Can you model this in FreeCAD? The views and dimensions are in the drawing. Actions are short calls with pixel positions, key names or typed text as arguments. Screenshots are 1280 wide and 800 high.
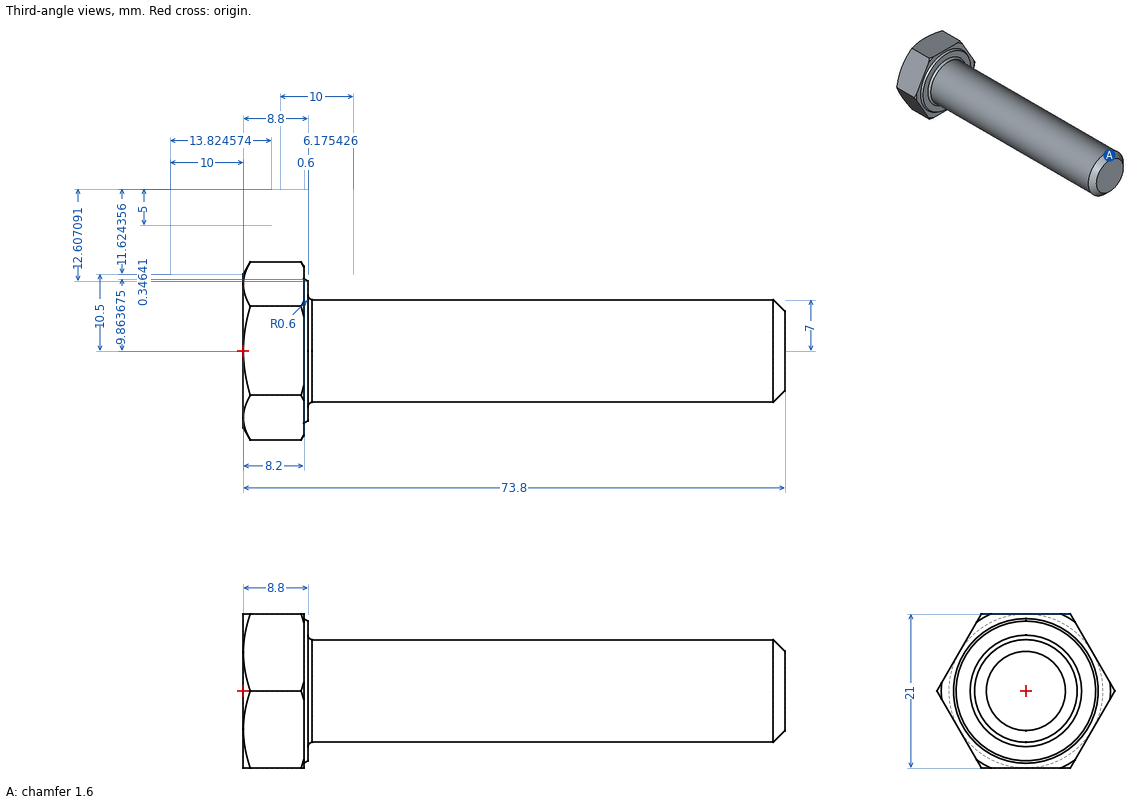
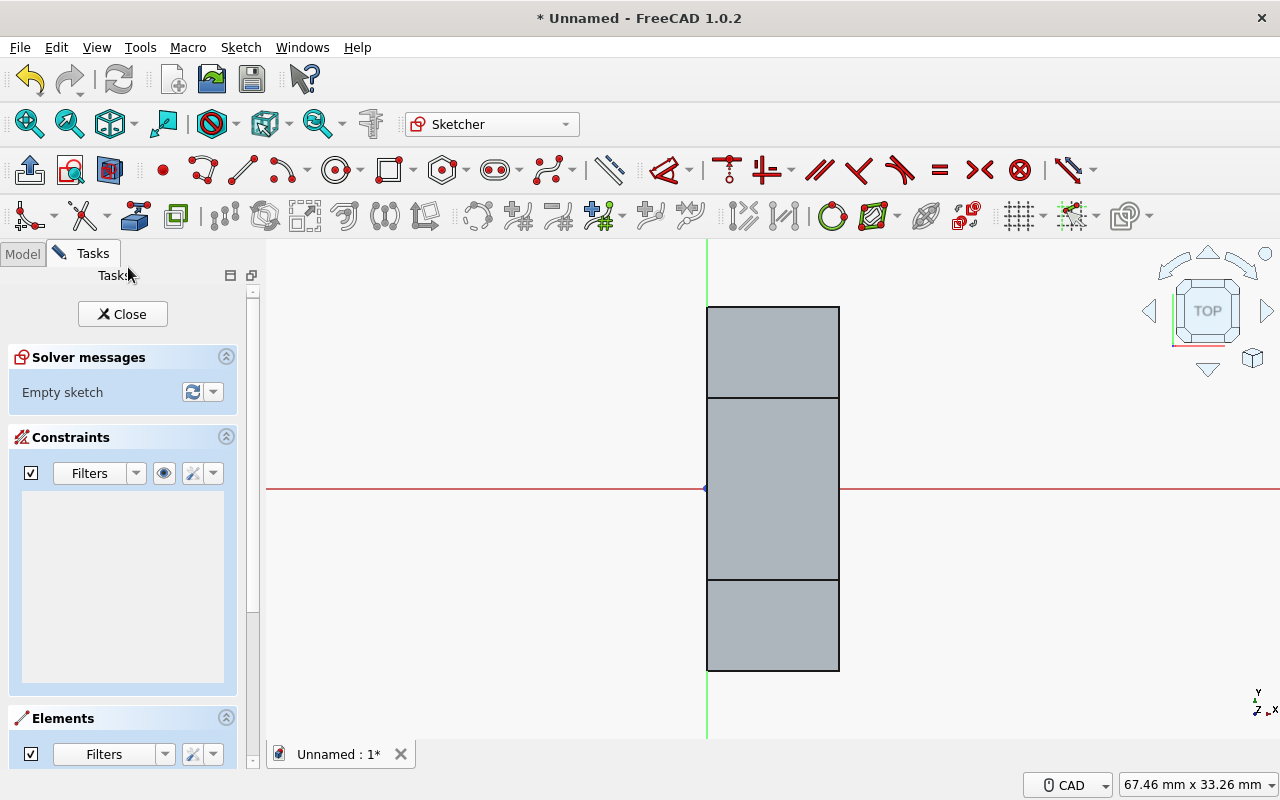
click(110, 170)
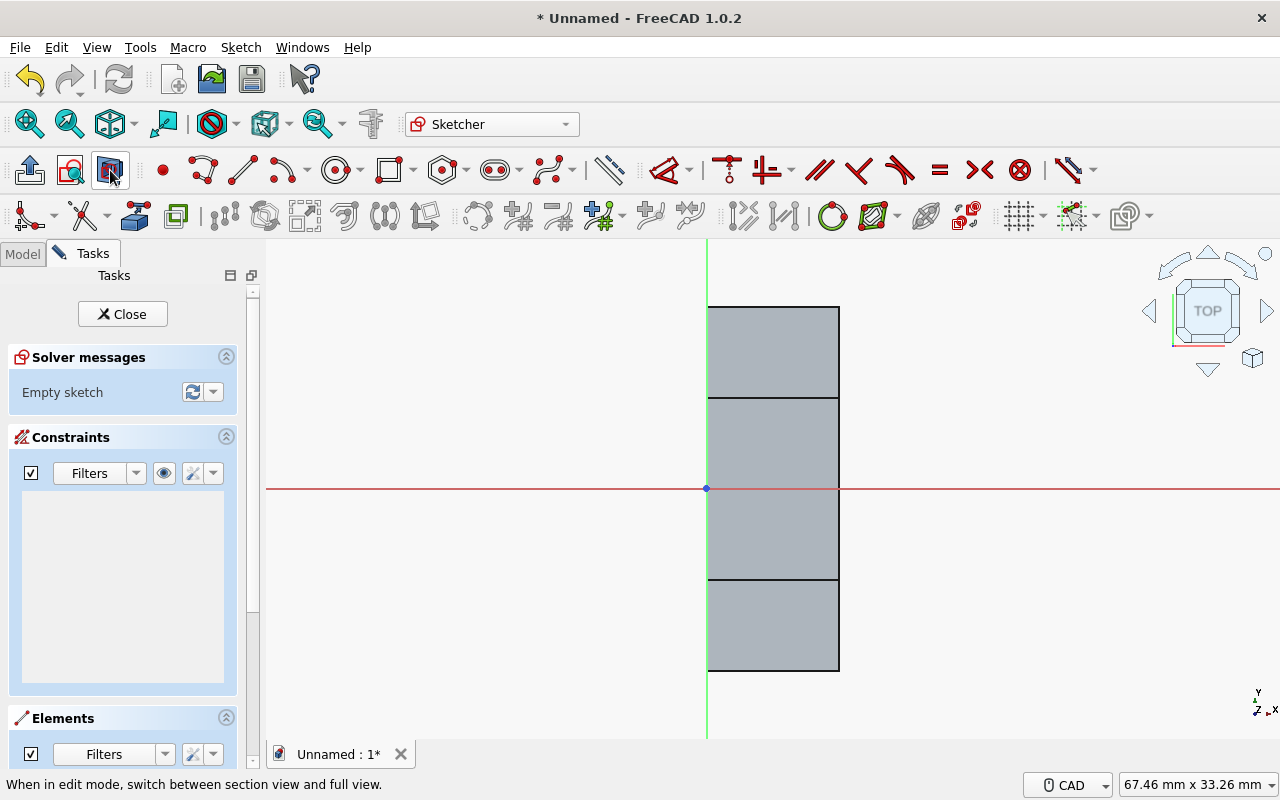
scroll(294, 532, down, 4)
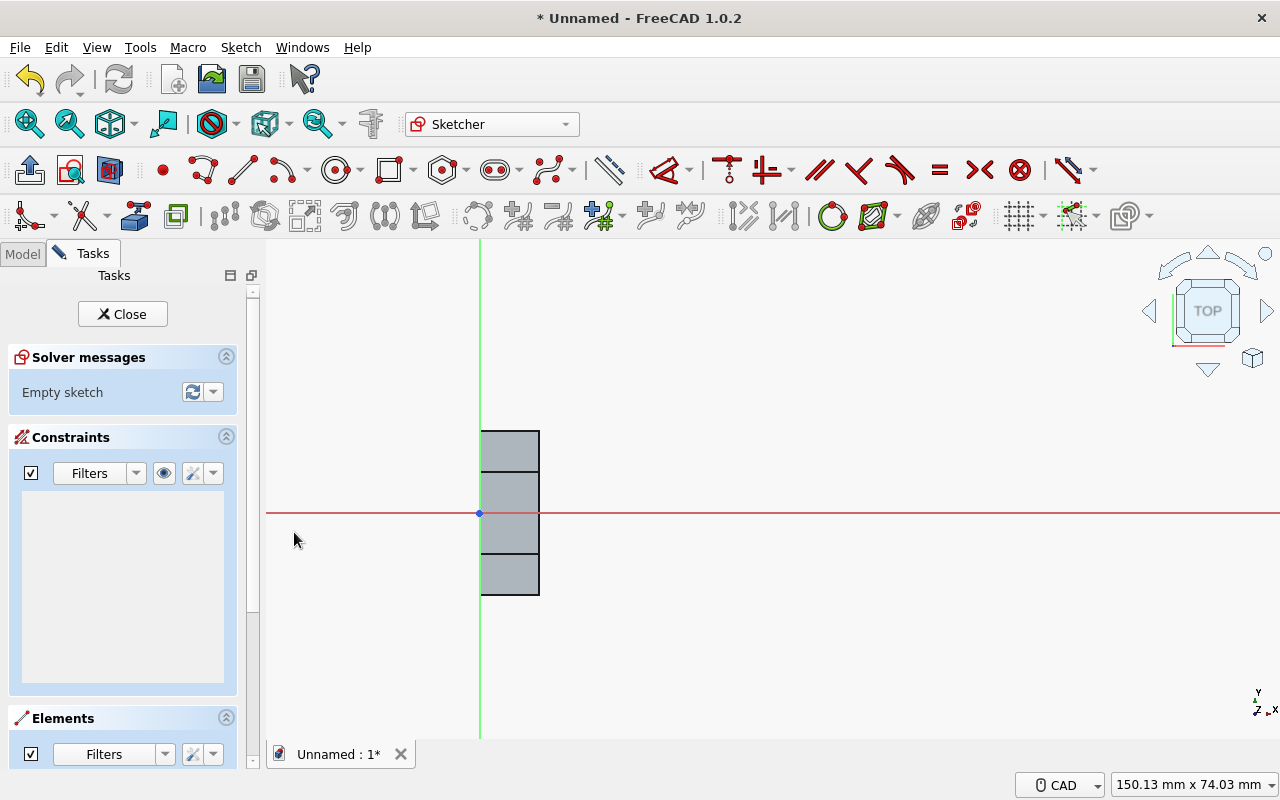
click(390, 170)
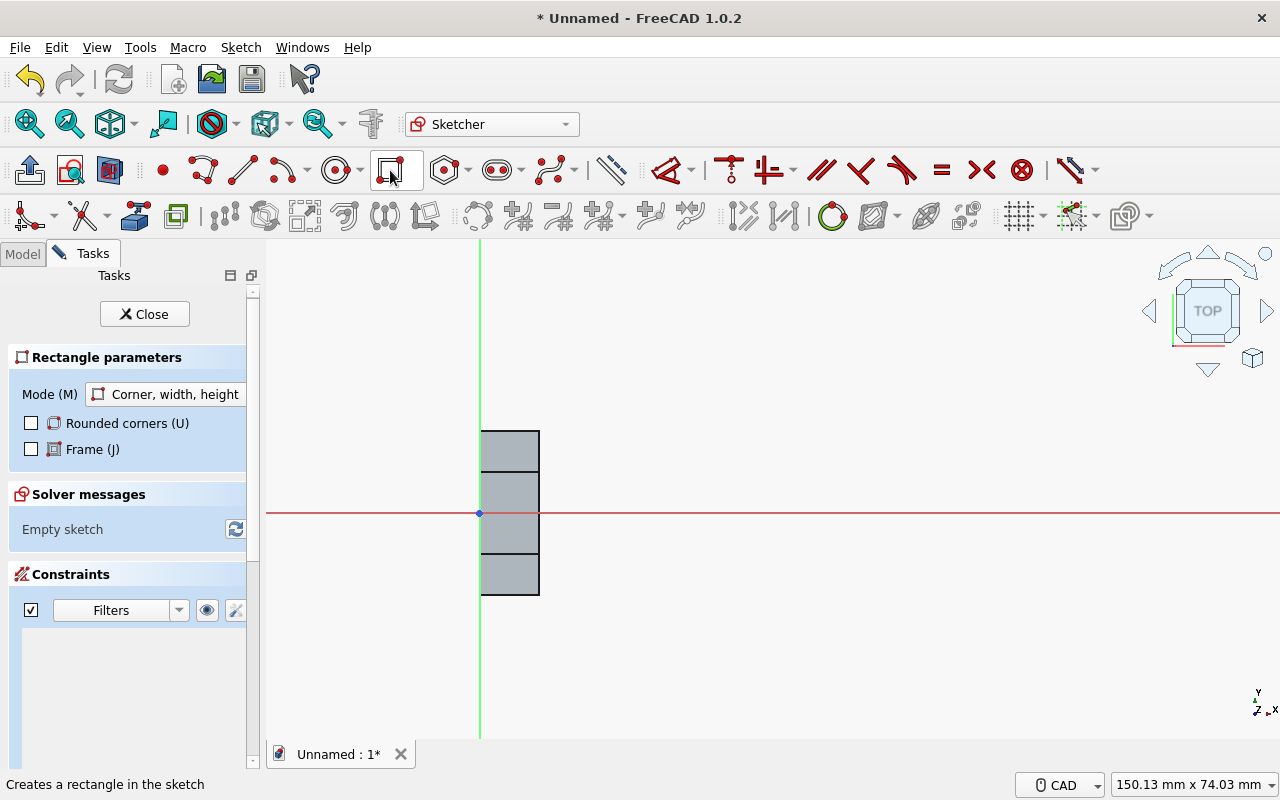
click(480, 513)
move(978, 466)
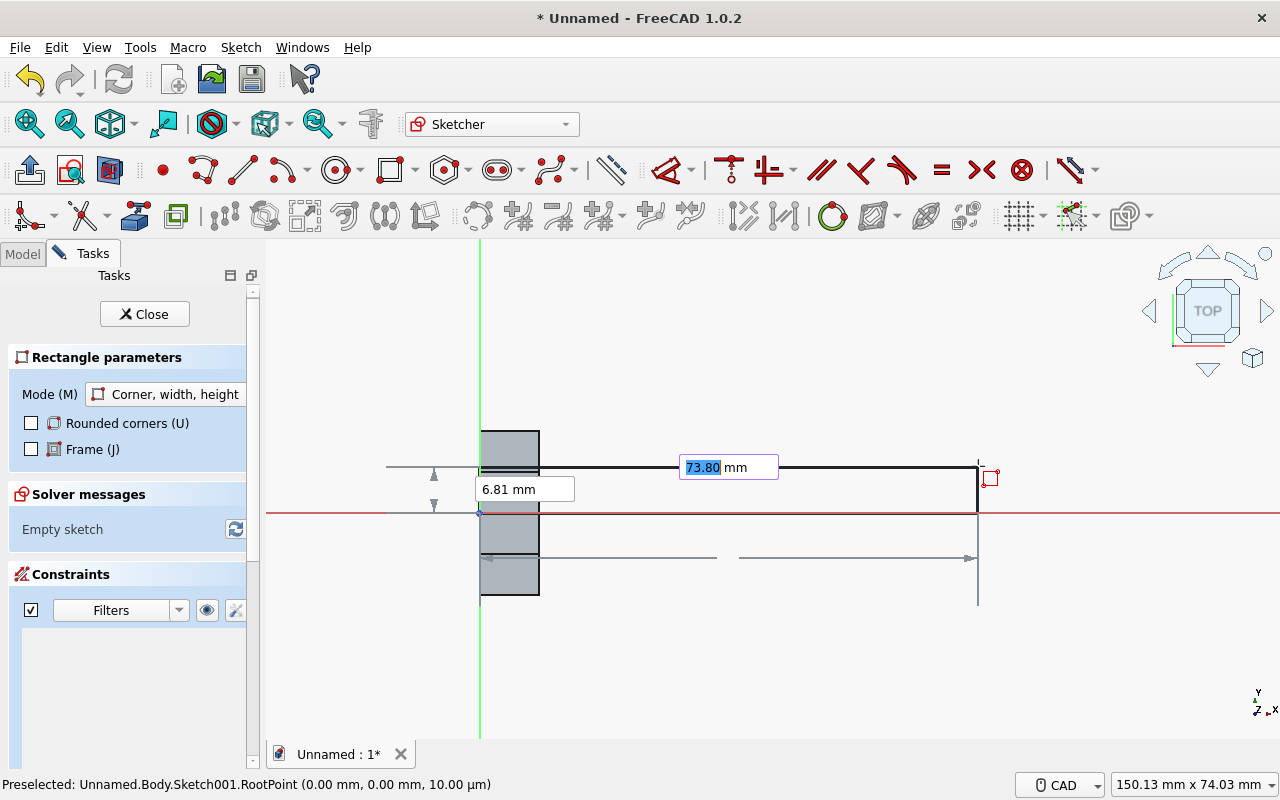
text(73.8)
key(Tab)
text(7)
key(Return)
key(Escape)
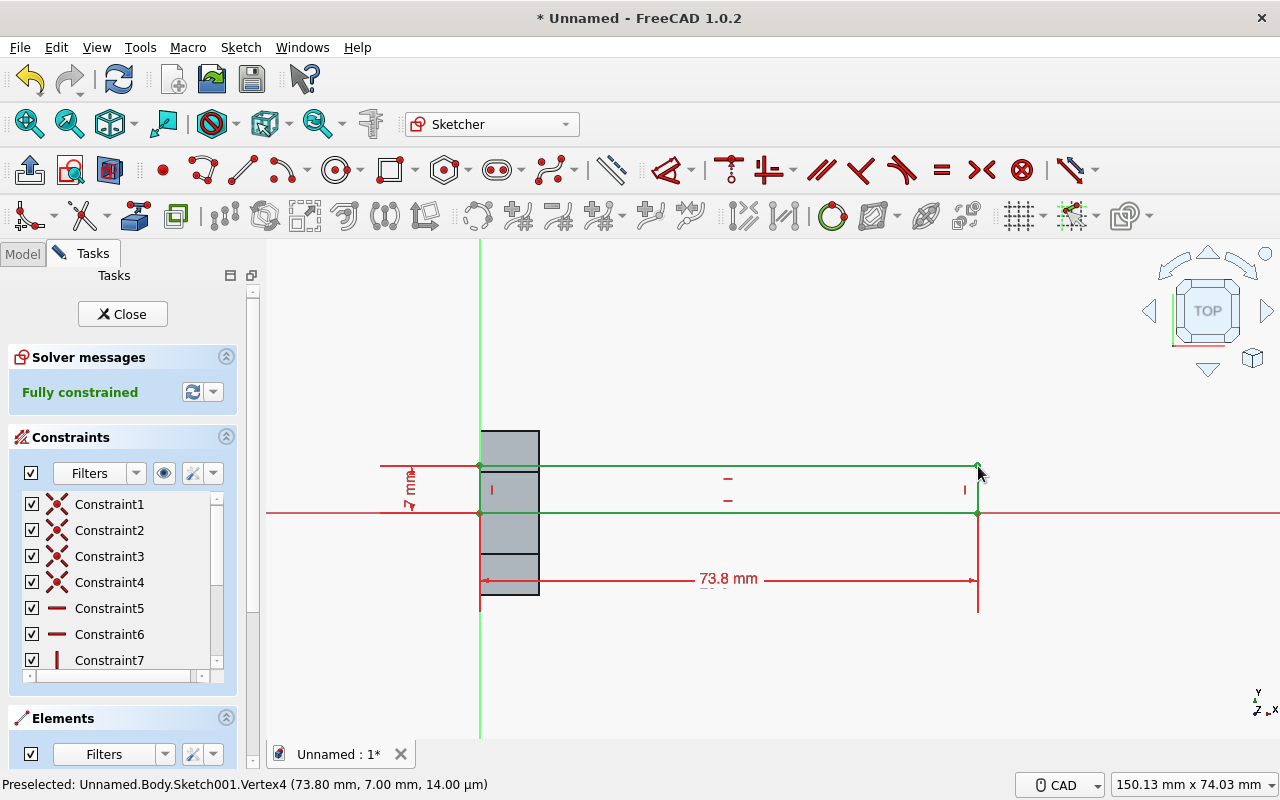
click(123, 314)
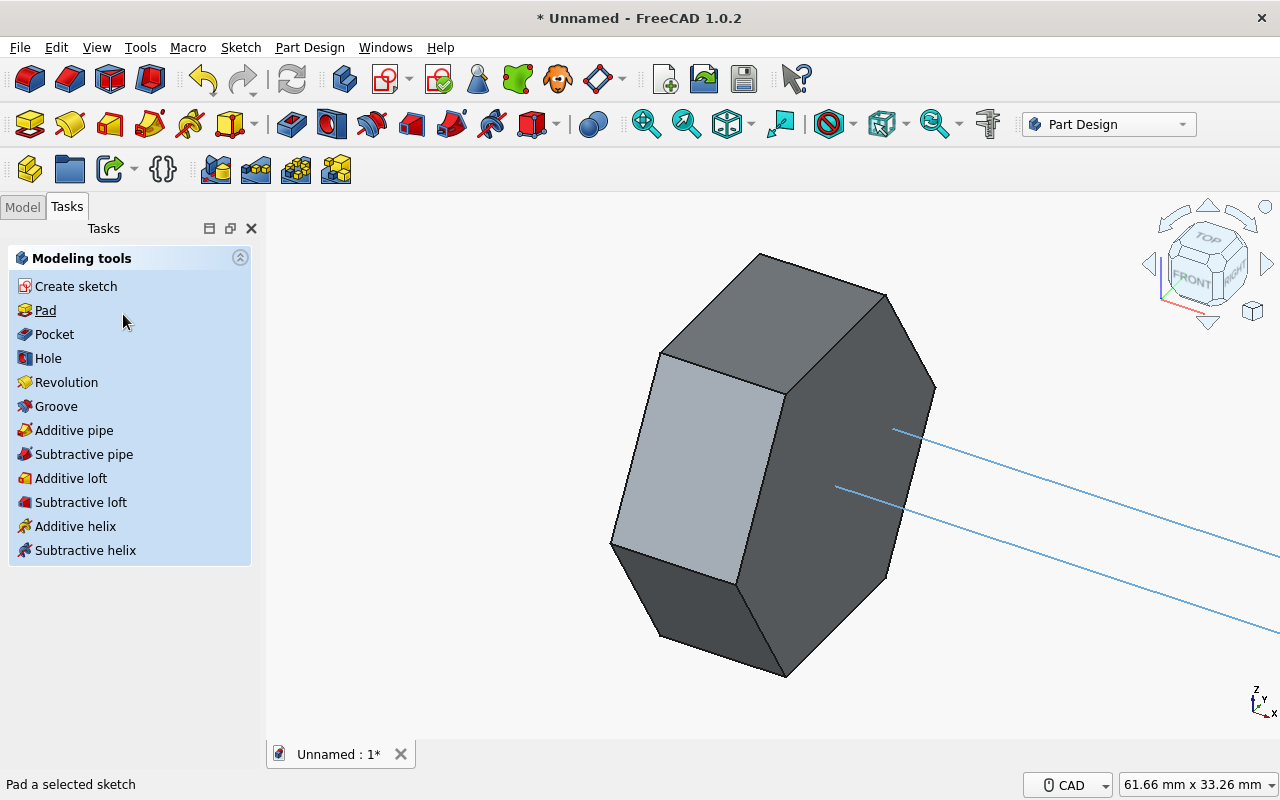
click(70, 124)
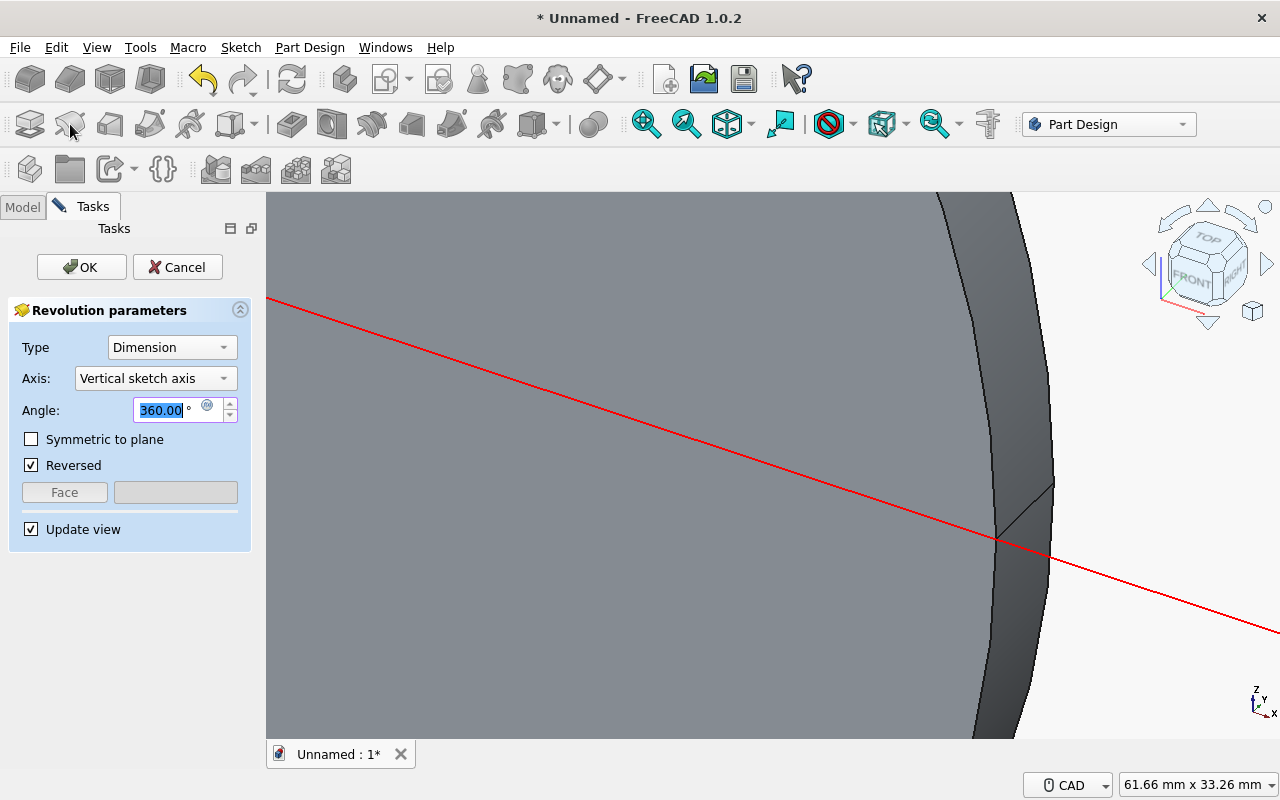
click(156, 378)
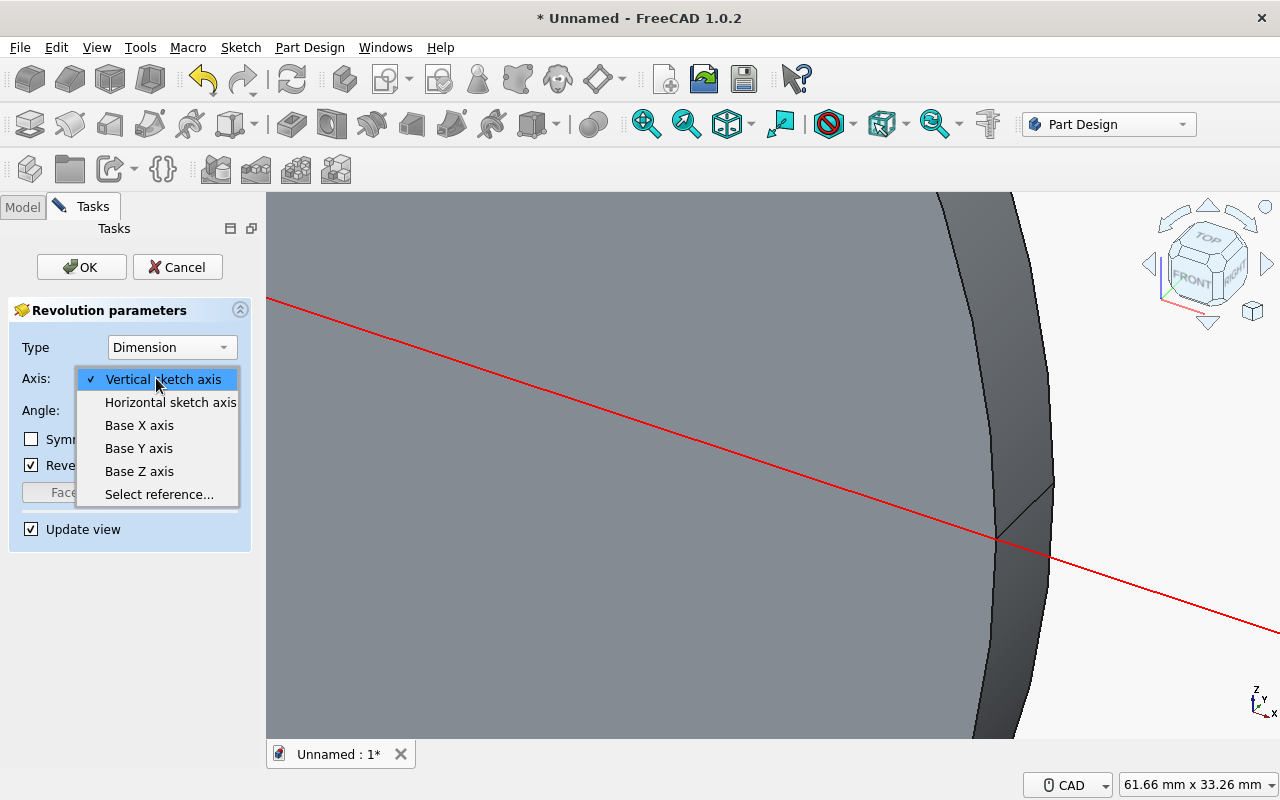
click(156, 402)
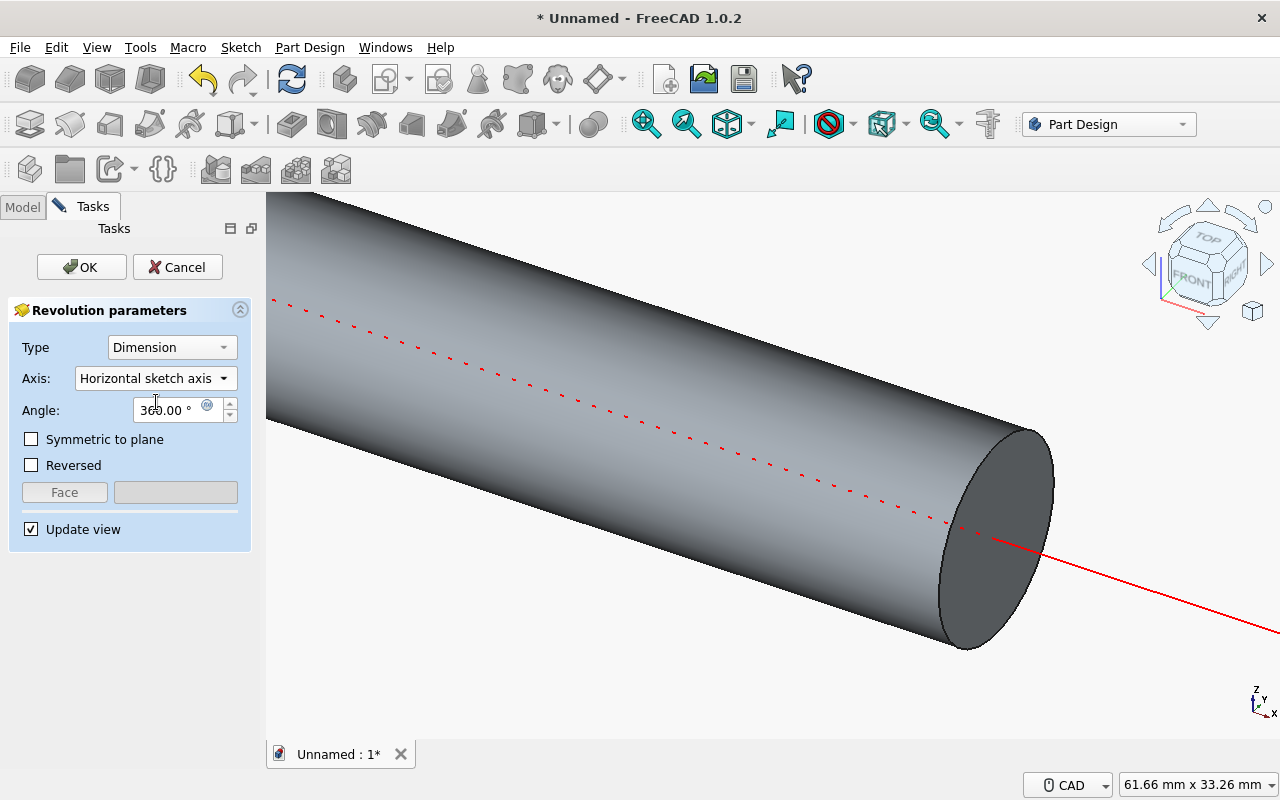
click(82, 267)